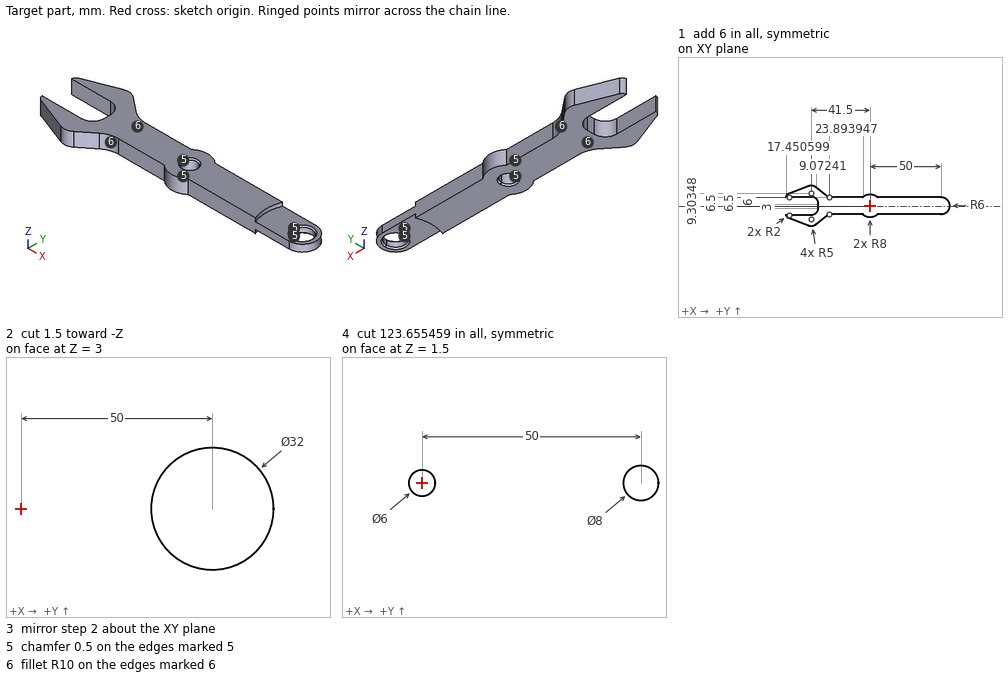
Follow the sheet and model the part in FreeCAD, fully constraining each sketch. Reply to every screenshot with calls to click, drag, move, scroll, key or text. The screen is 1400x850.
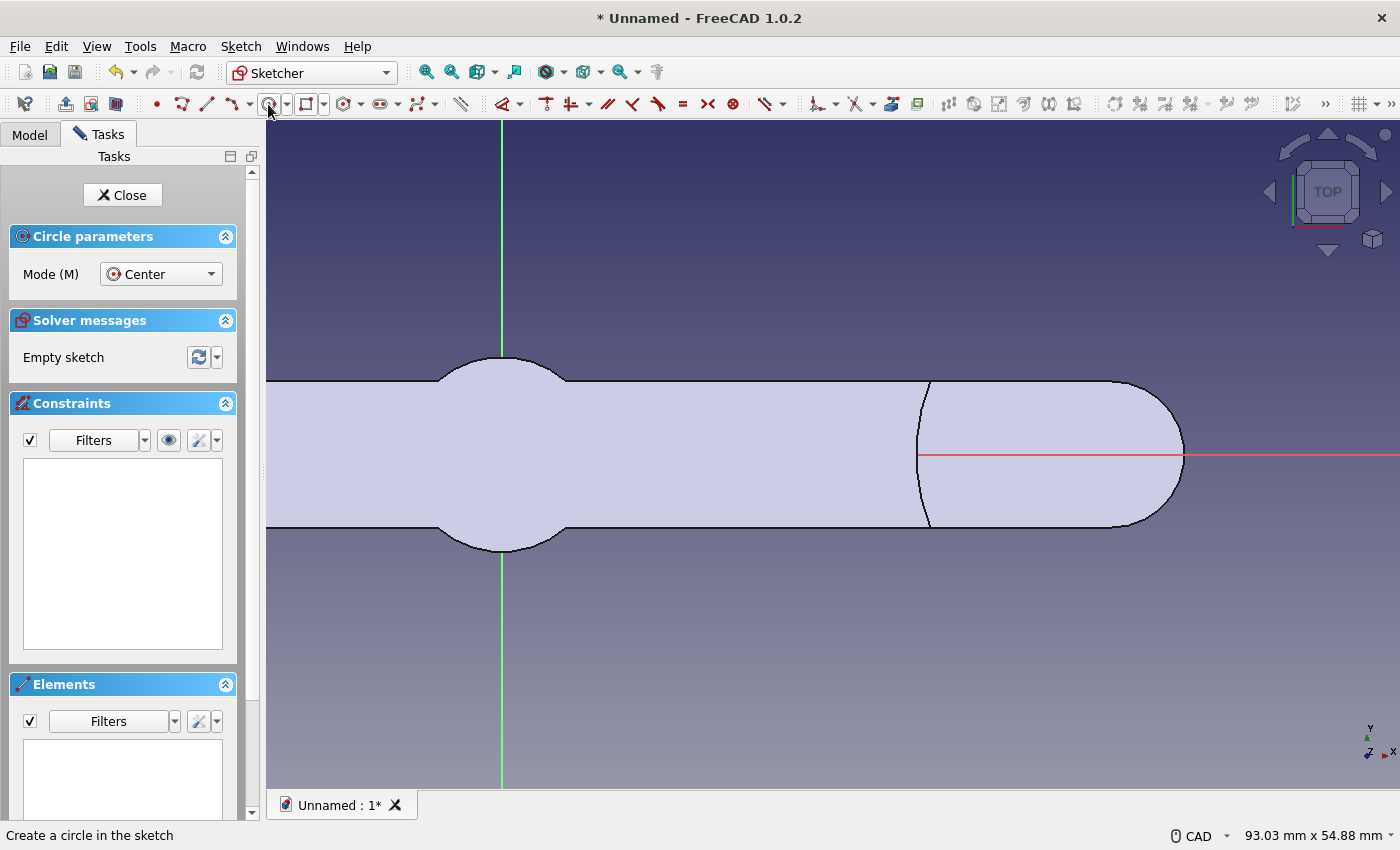
click(1111, 454)
move(1146, 420)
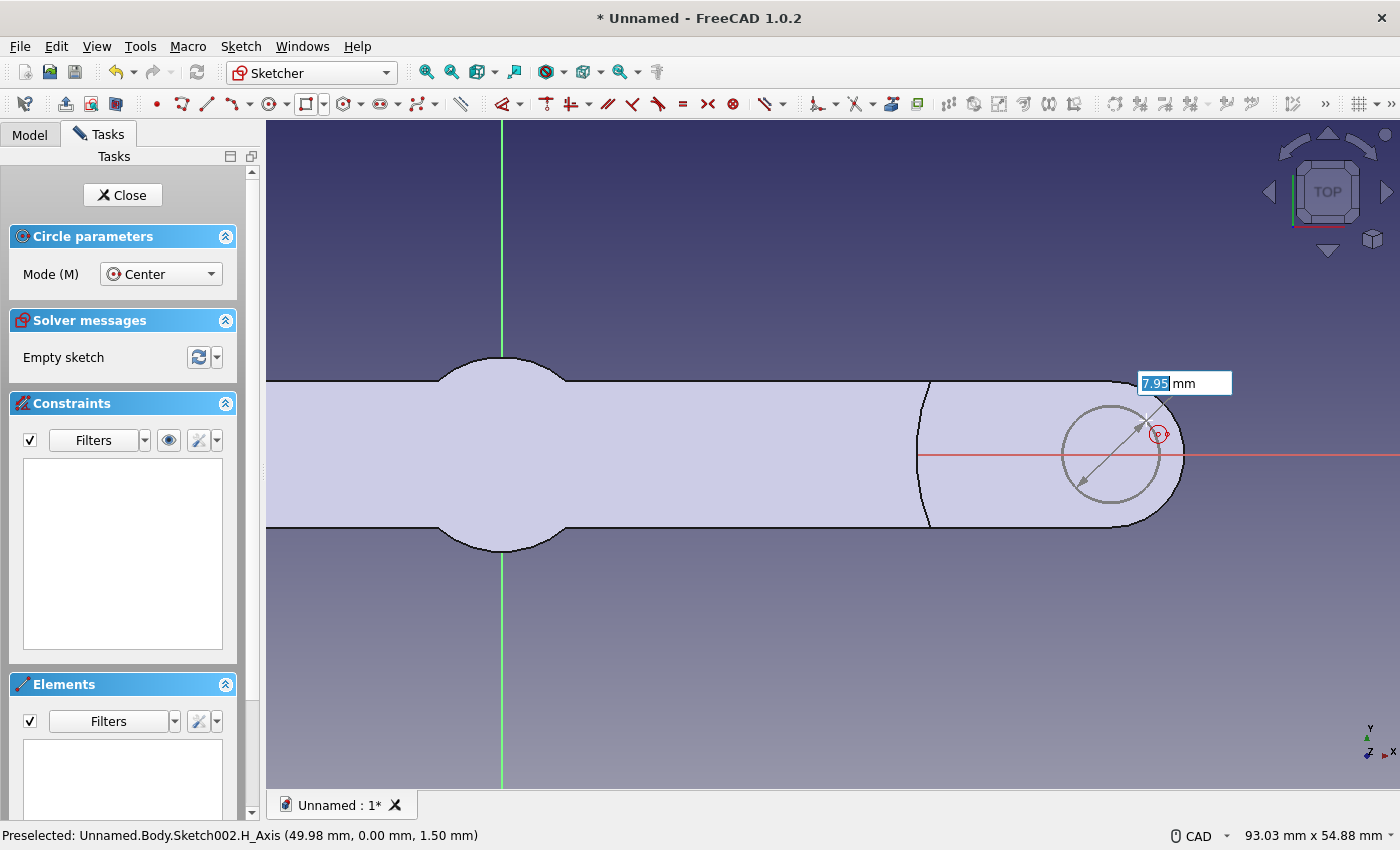
text(8)
key(Return)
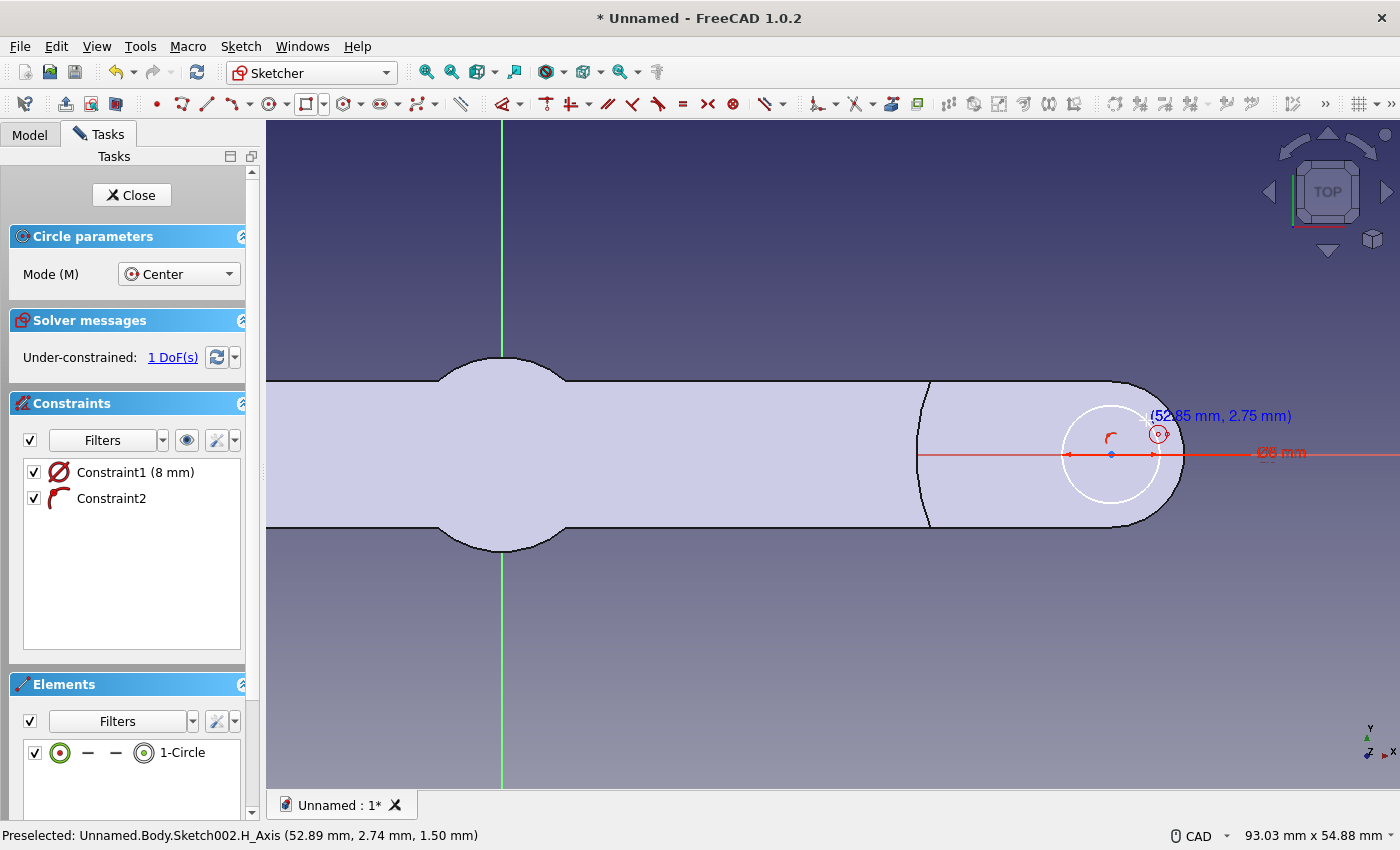
click(502, 454)
move(528, 429)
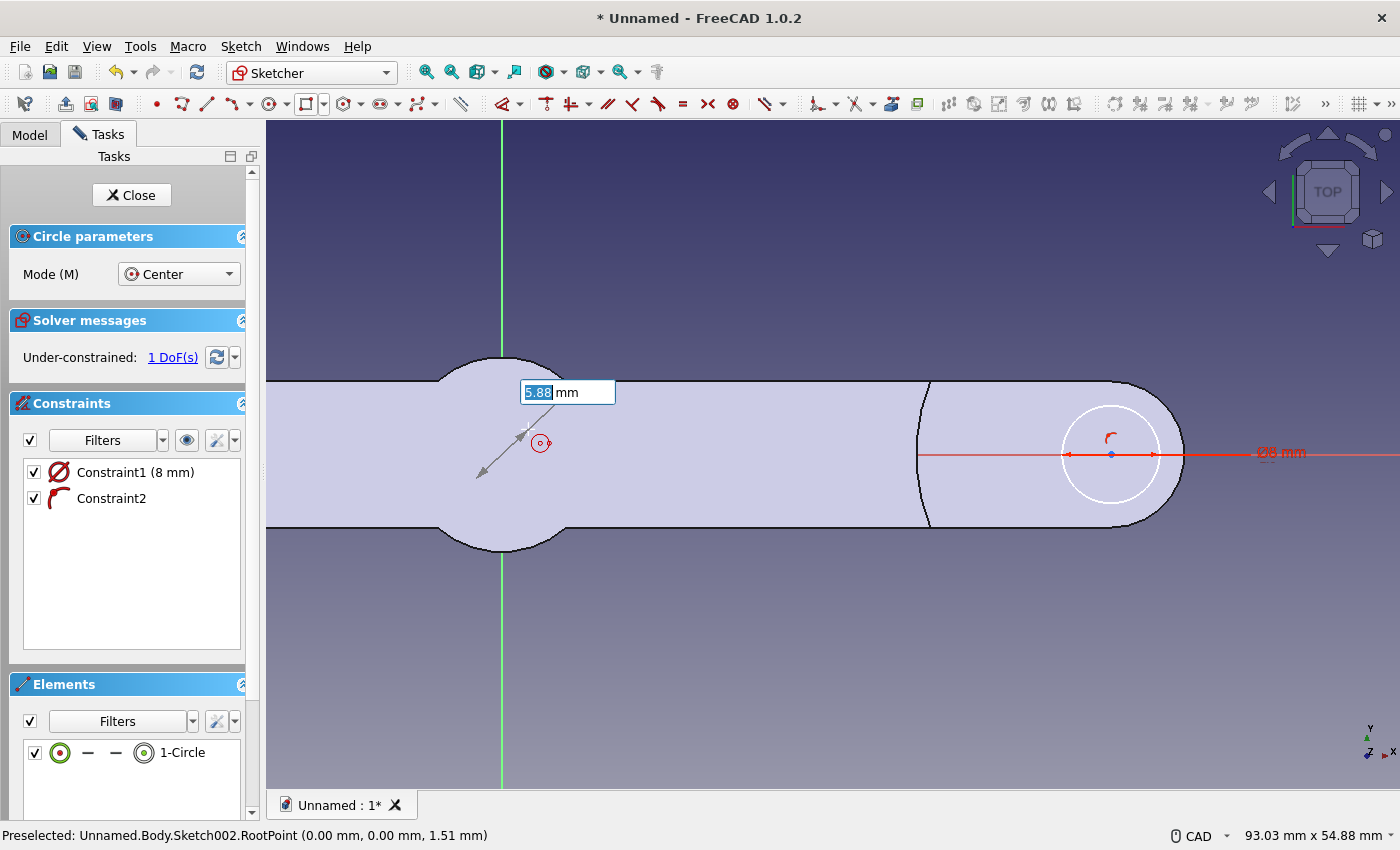
text(6)
key(Return)
key(Escape)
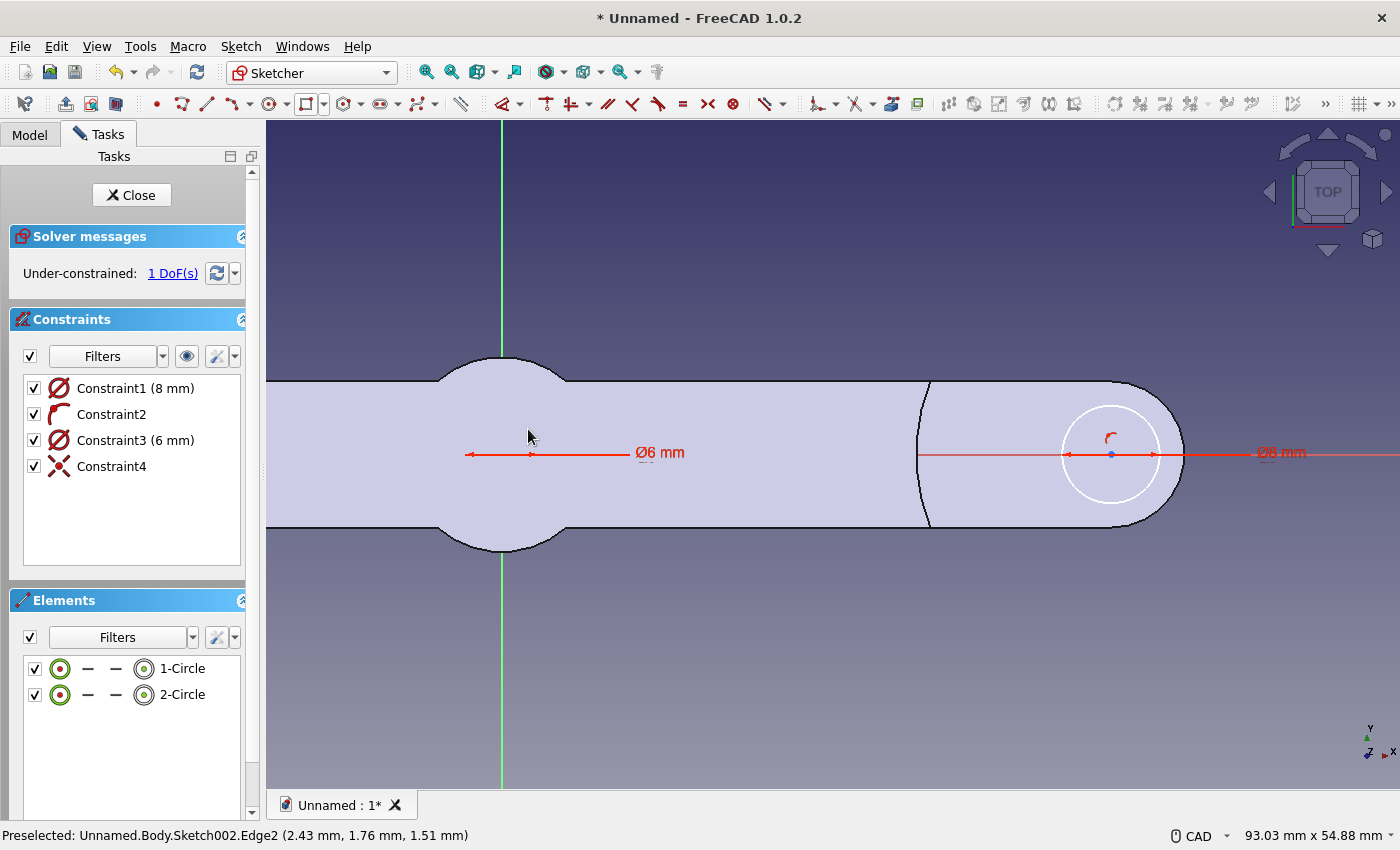
click(502, 104)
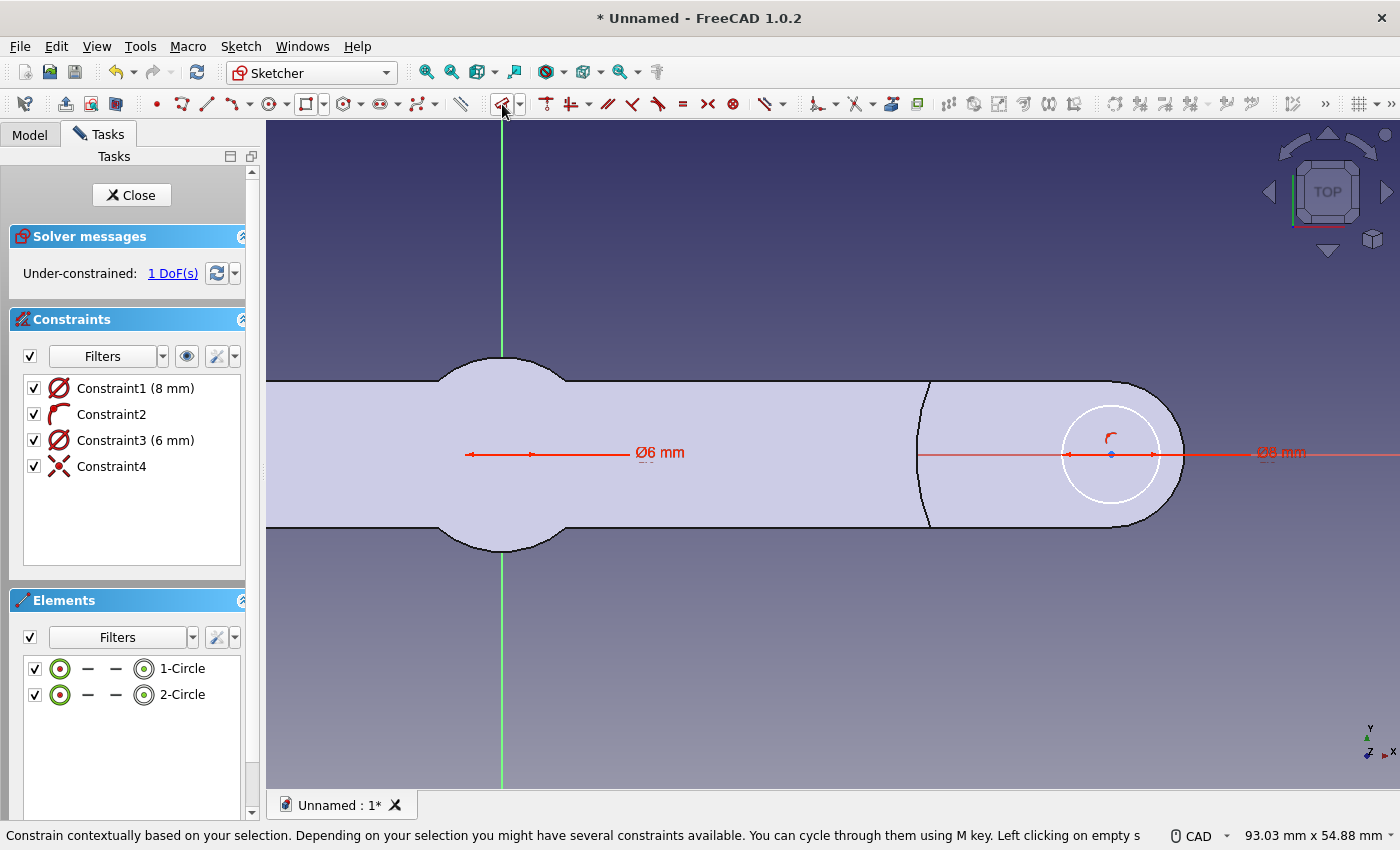
click(1111, 454)
click(806, 488)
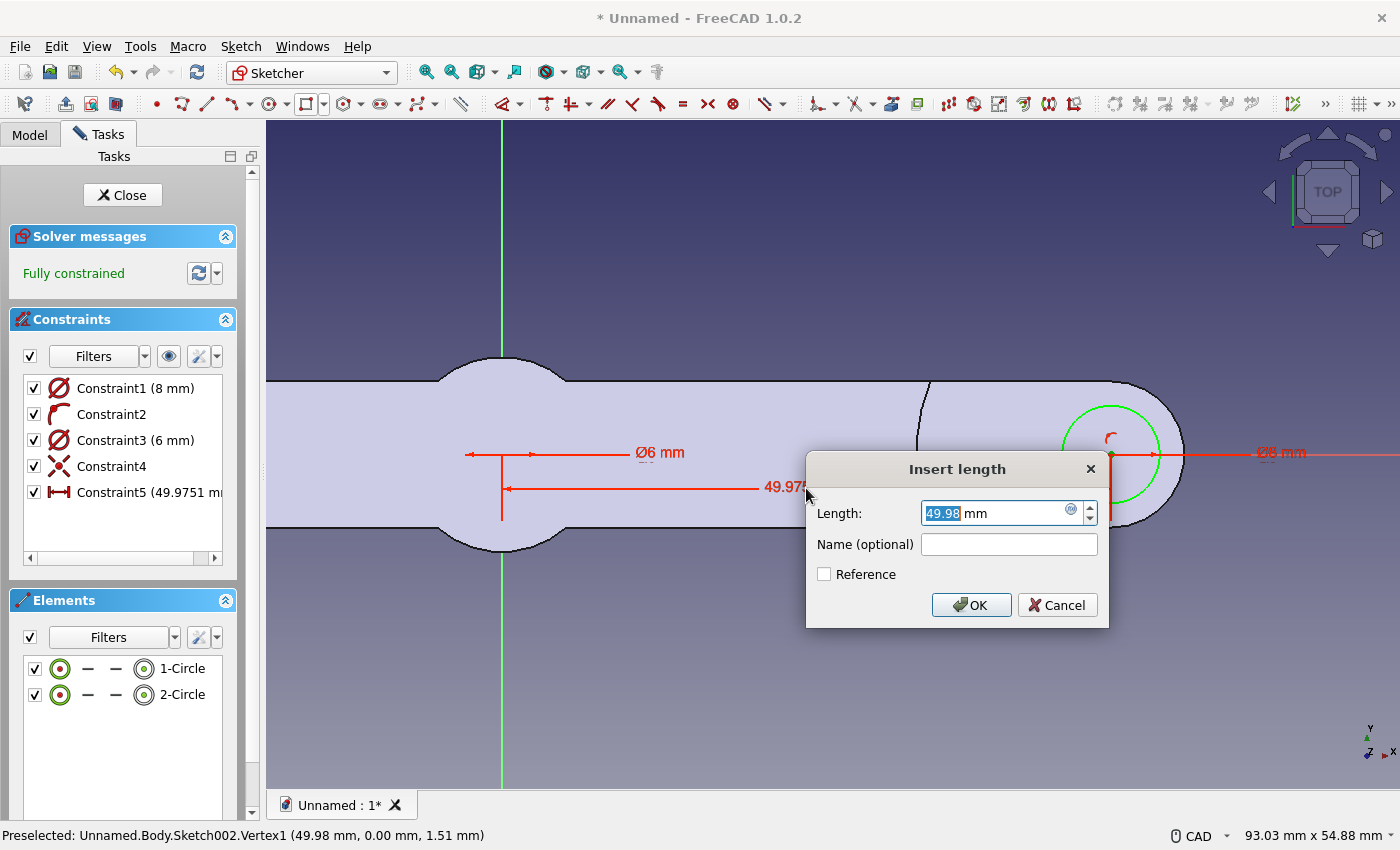
text(50)
key(Return)
key(Escape)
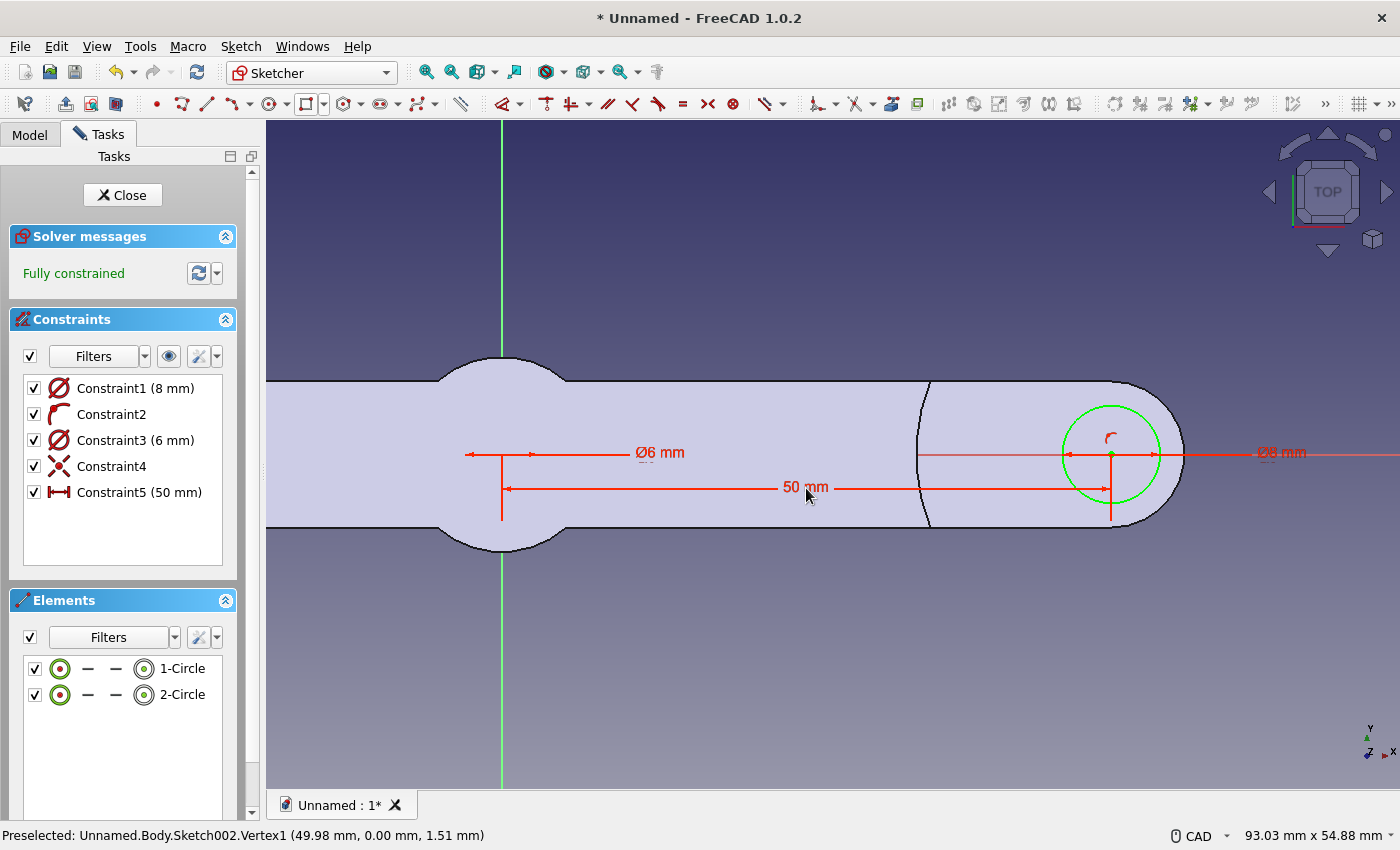
click(123, 195)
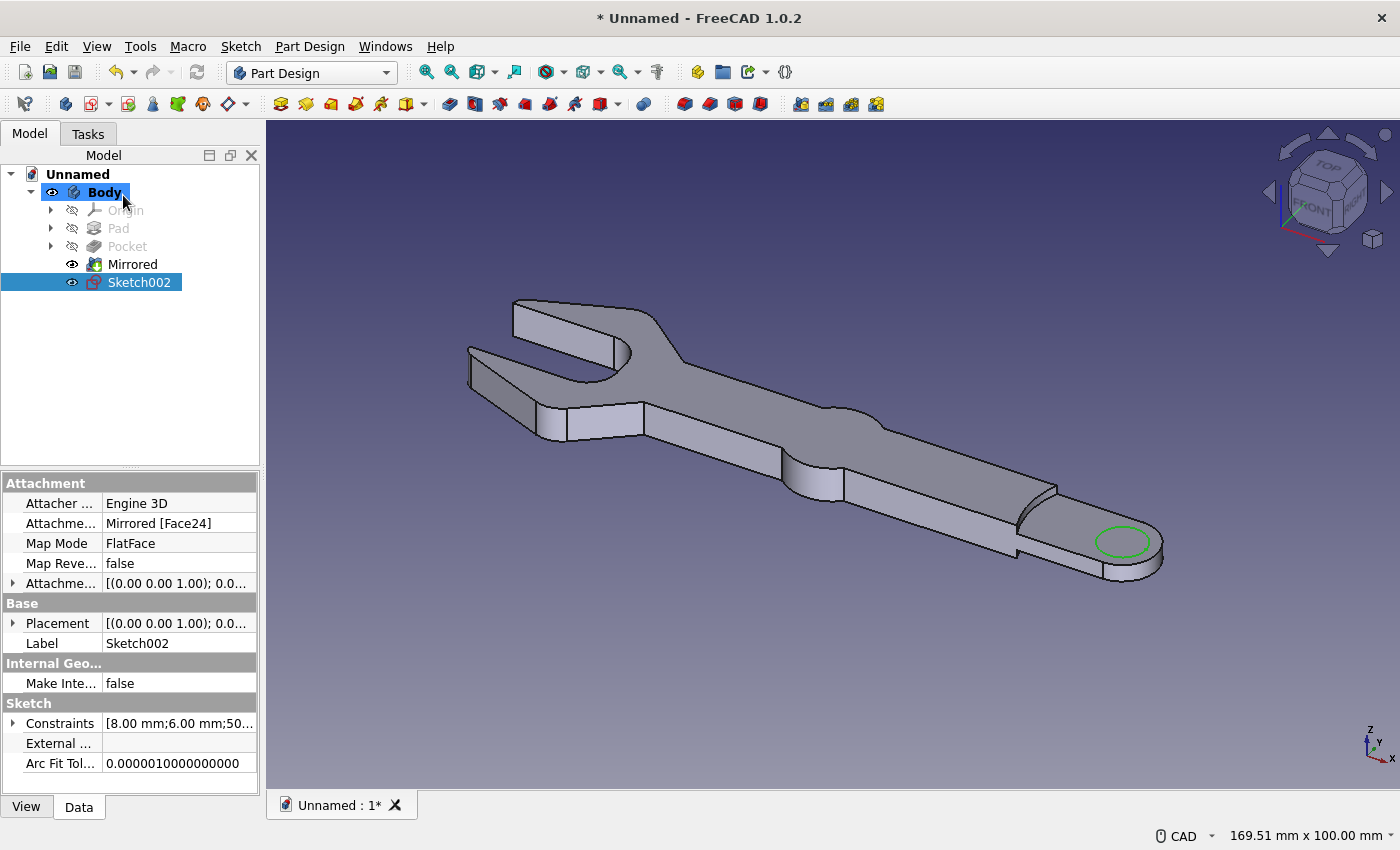
click(450, 104)